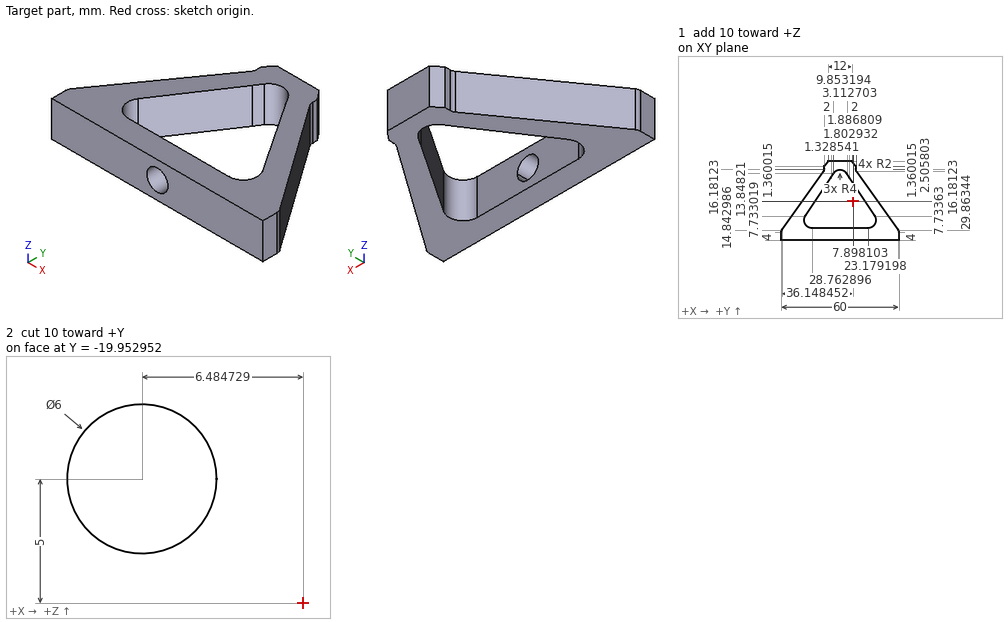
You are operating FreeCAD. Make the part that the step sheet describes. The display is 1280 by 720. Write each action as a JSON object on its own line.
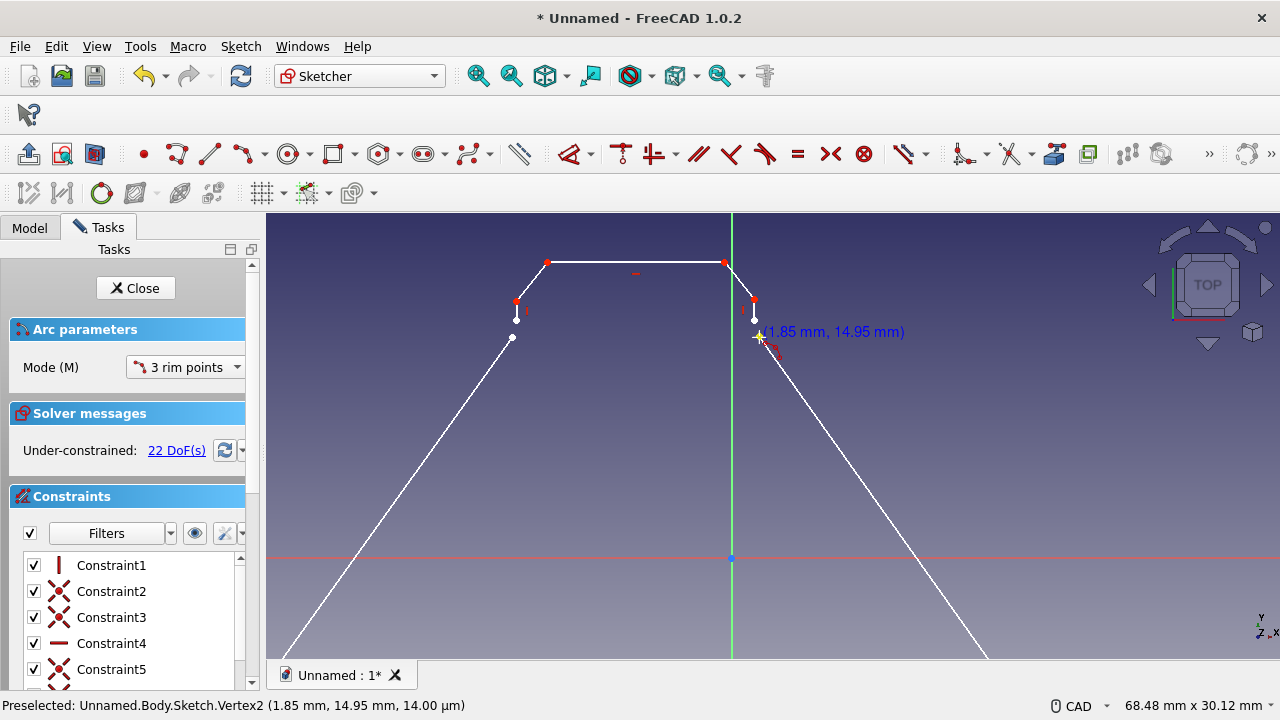
{"action": "scroll", "coordinate": [754, 319], "scroll_direction": "up", "scroll_amount": 3}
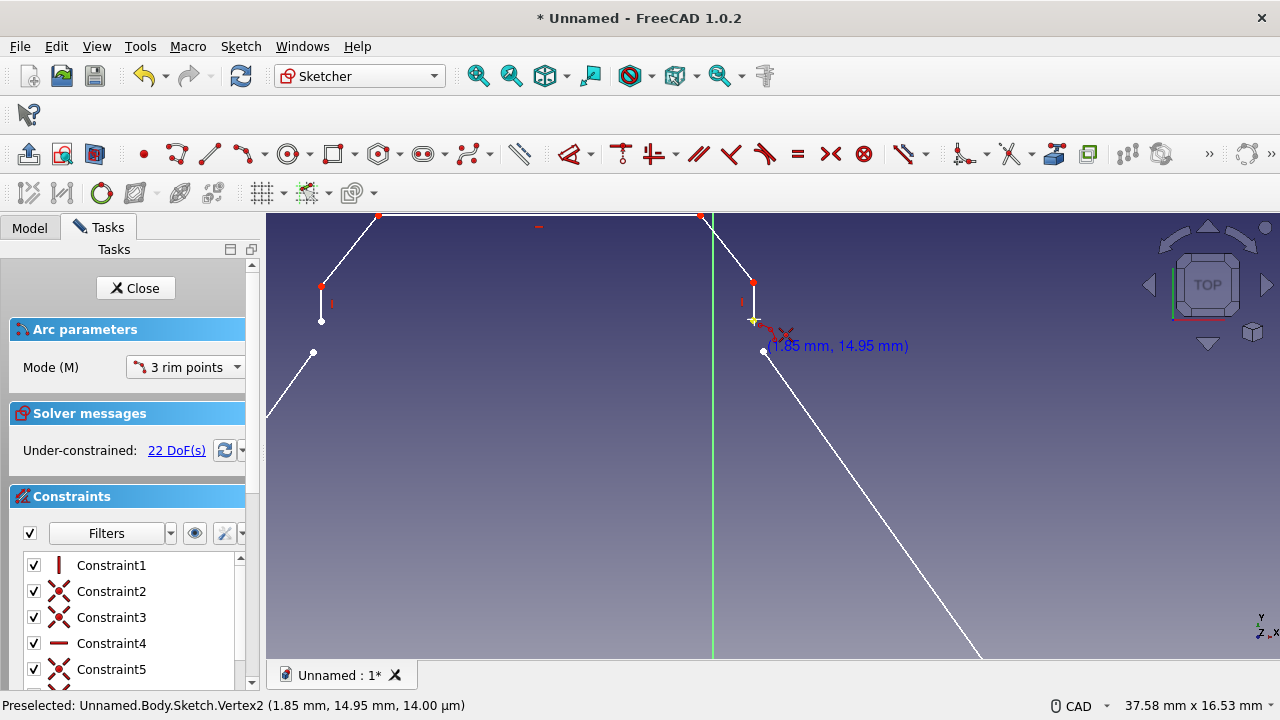
{"action": "left_click", "coordinate": [754, 321]}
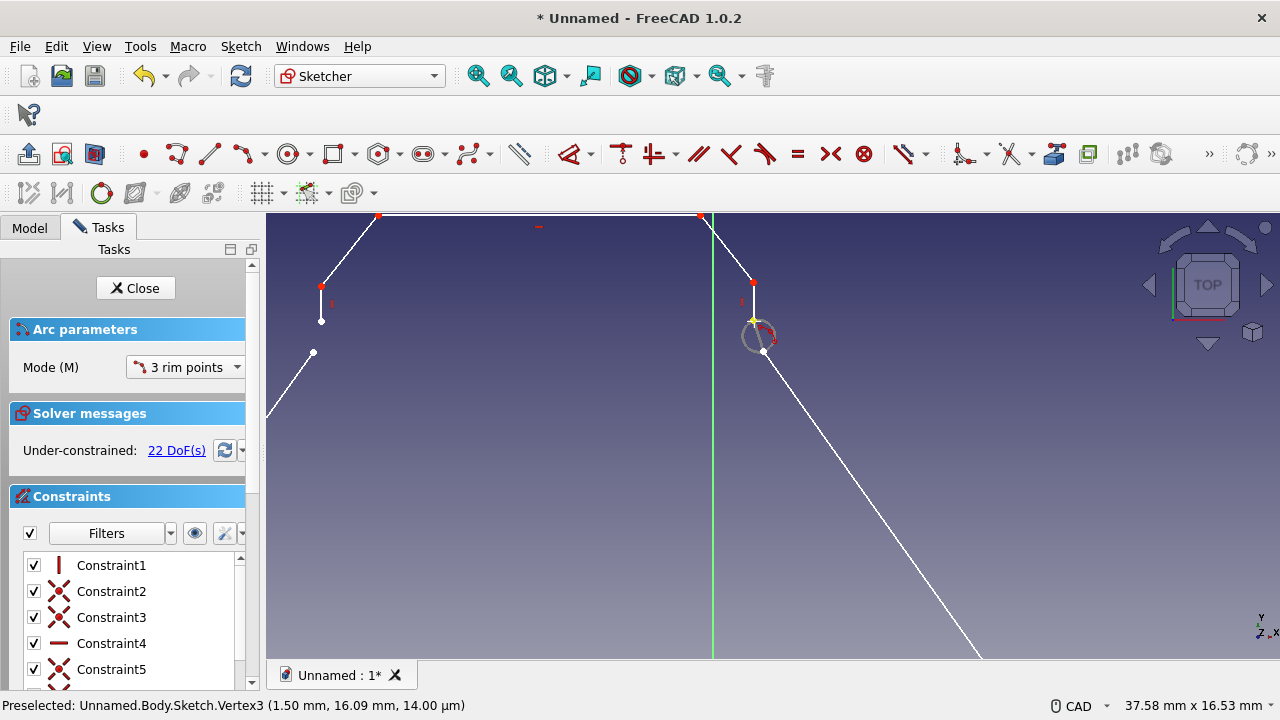
{"action": "scroll", "coordinate": [757, 335], "scroll_direction": "up", "scroll_amount": 10}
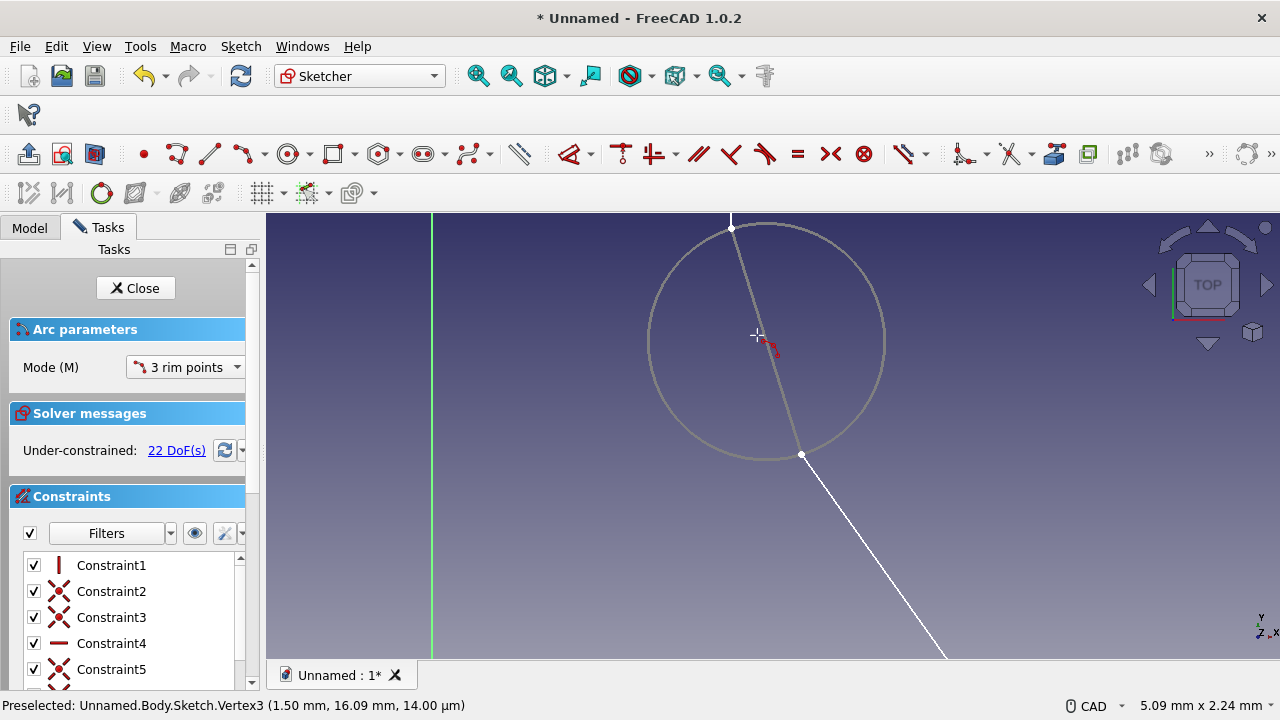
{"action": "left_click", "coordinate": [753, 331]}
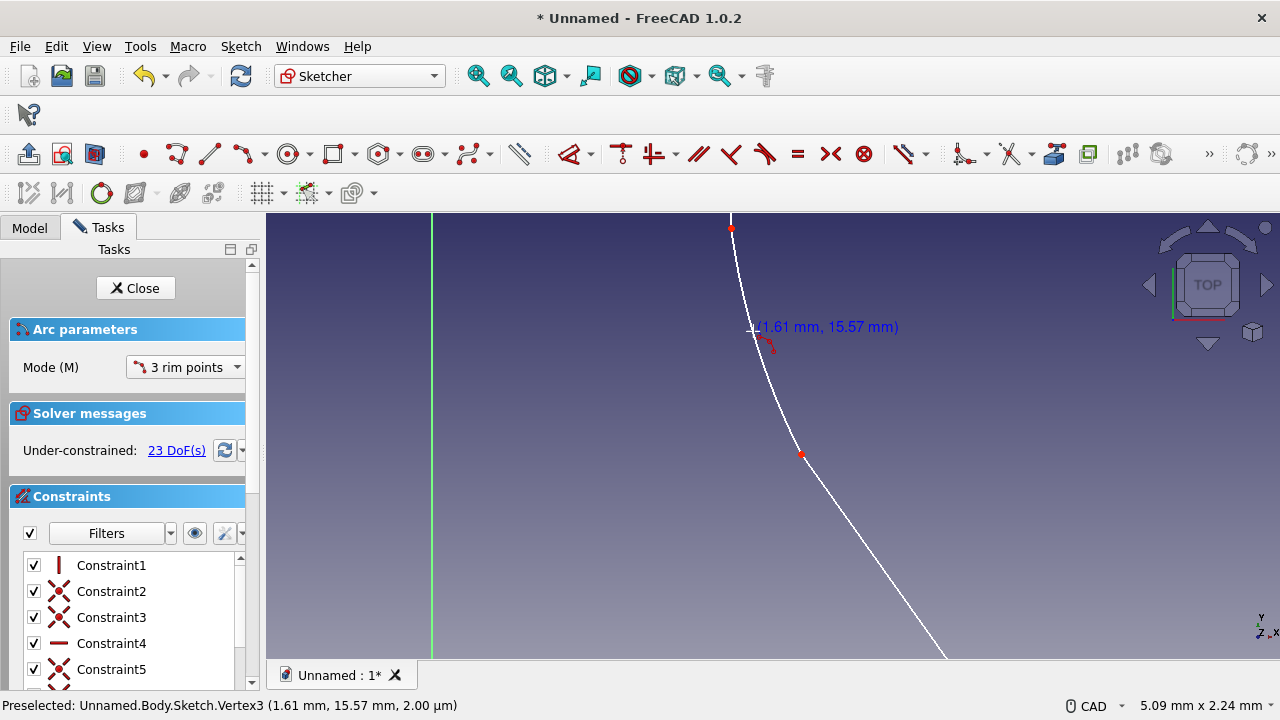
{"action": "scroll", "coordinate": [771, 309], "scroll_direction": "down", "scroll_amount": 16}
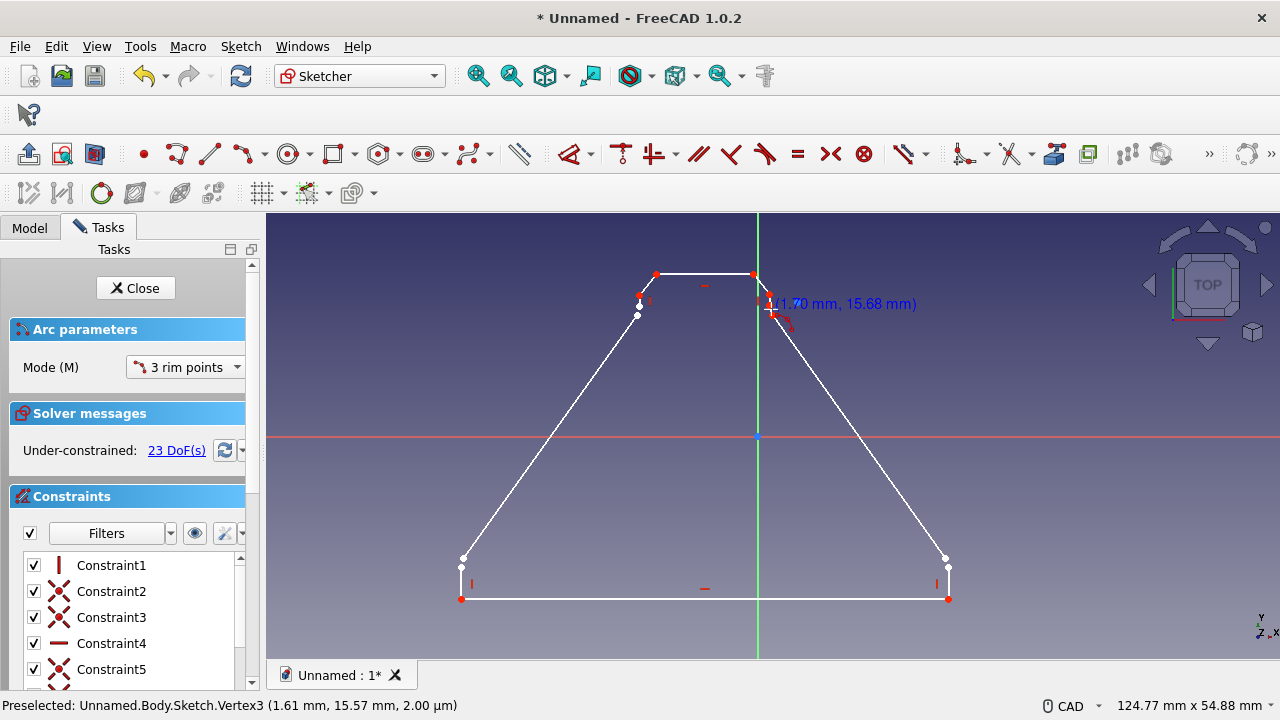
{"action": "scroll", "coordinate": [640, 305], "scroll_direction": "up", "scroll_amount": 6}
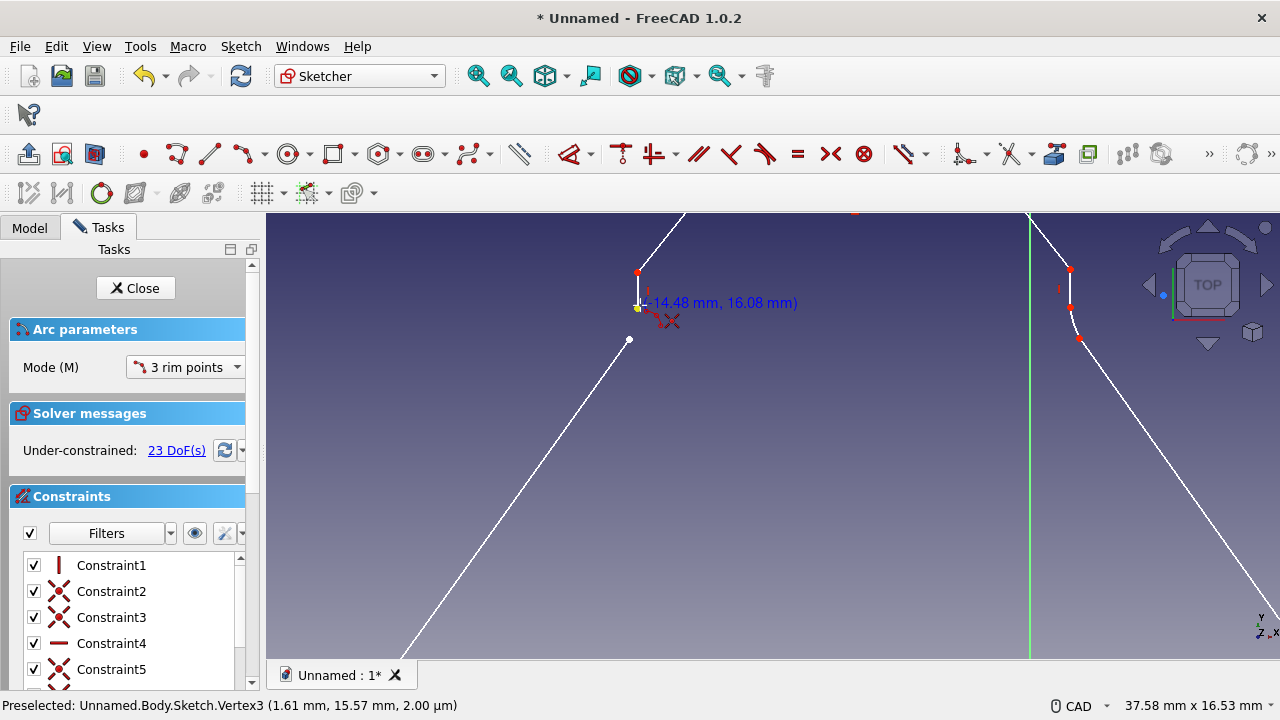
{"action": "left_click", "coordinate": [638, 308]}
{"action": "left_click", "coordinate": [630, 339]}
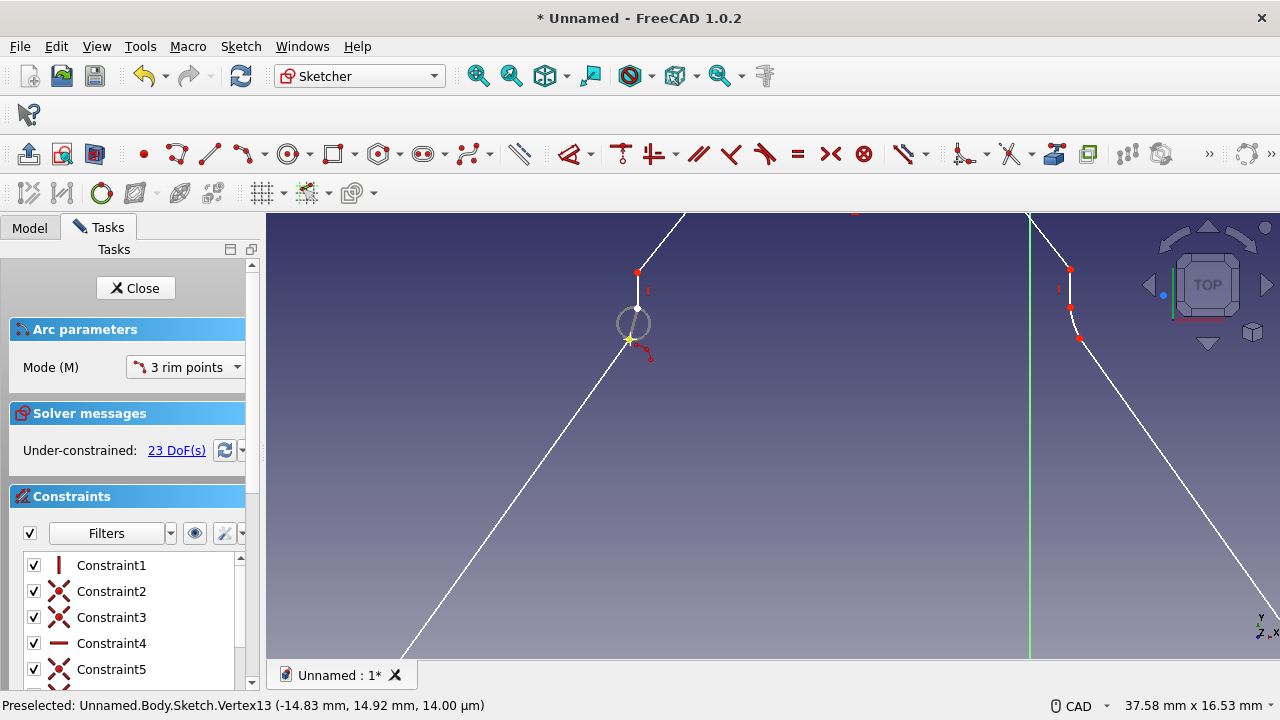
{"action": "scroll", "coordinate": [636, 321], "scroll_direction": "up", "scroll_amount": 10}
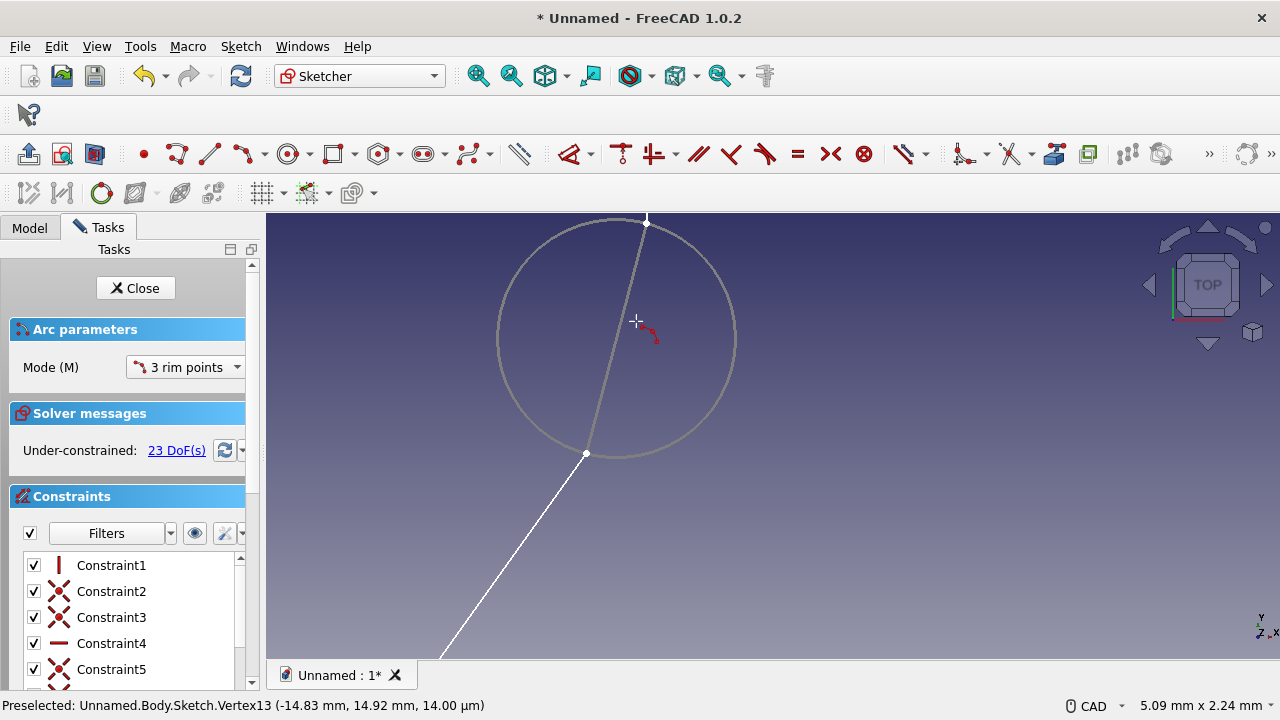
{"action": "left_click", "coordinate": [637, 323]}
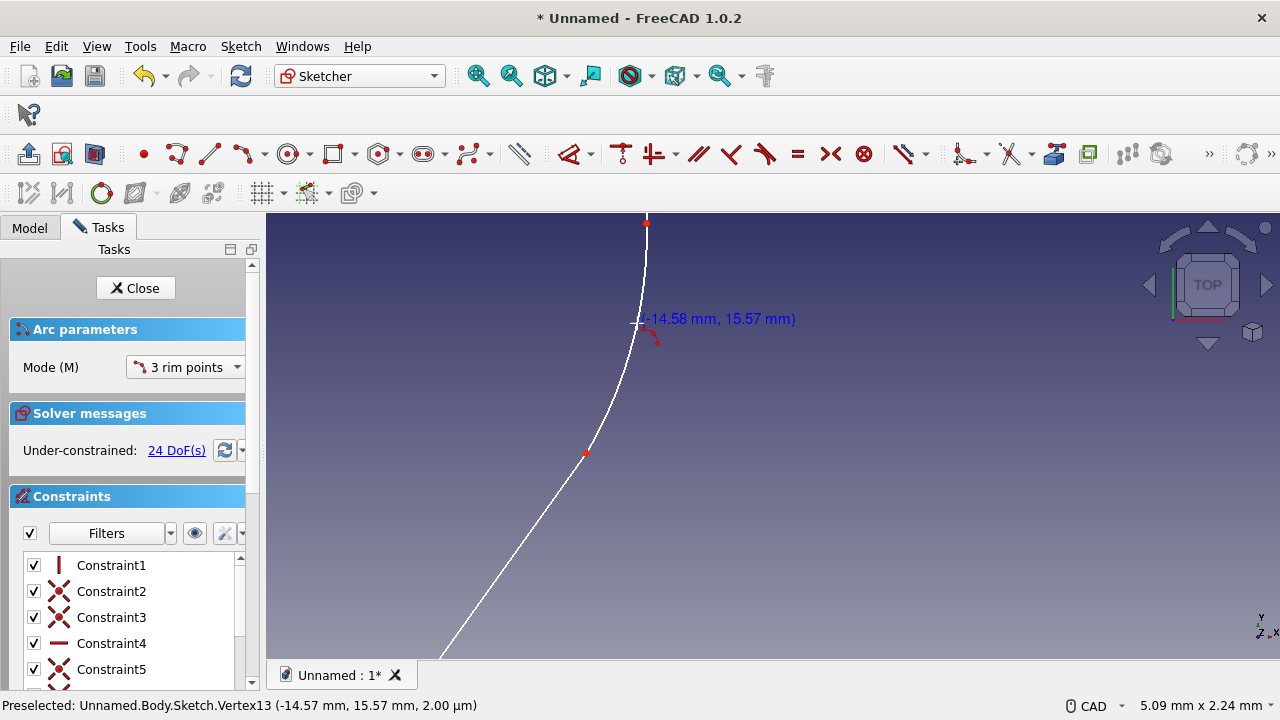
{"action": "scroll", "coordinate": [639, 309], "scroll_direction": "down", "scroll_amount": 16}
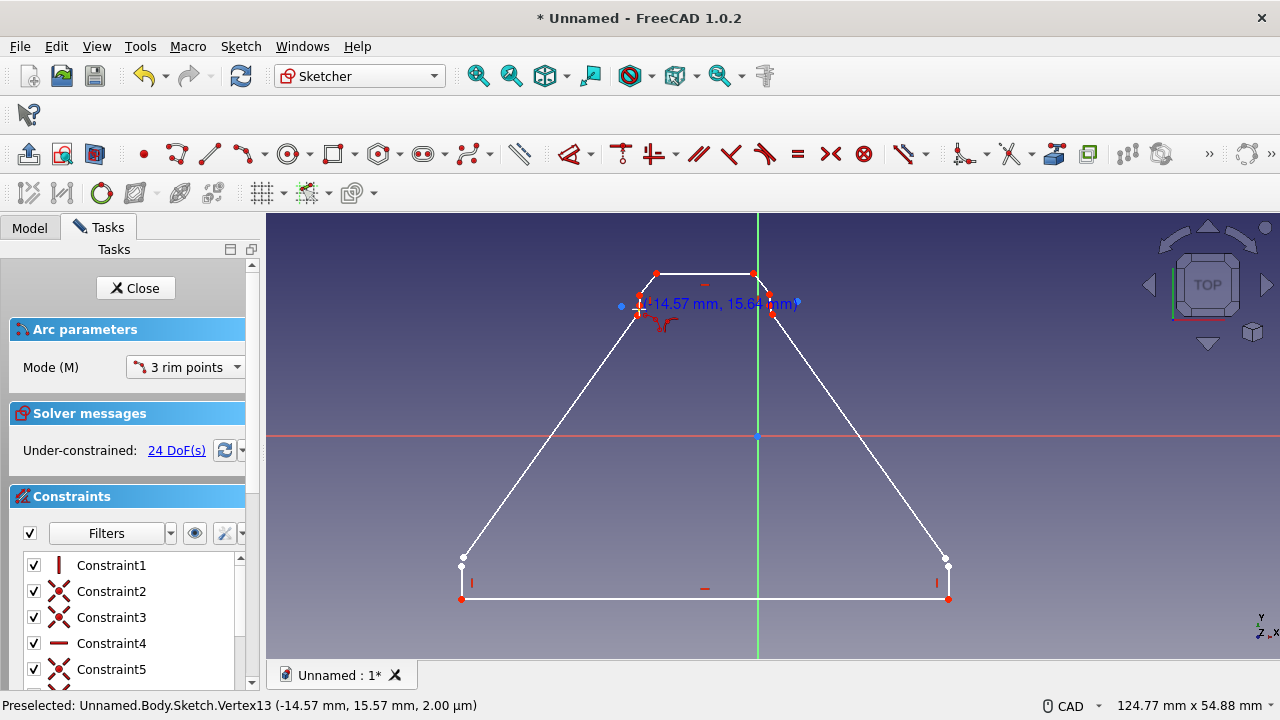
{"action": "scroll", "coordinate": [464, 557], "scroll_direction": "up", "scroll_amount": 3}